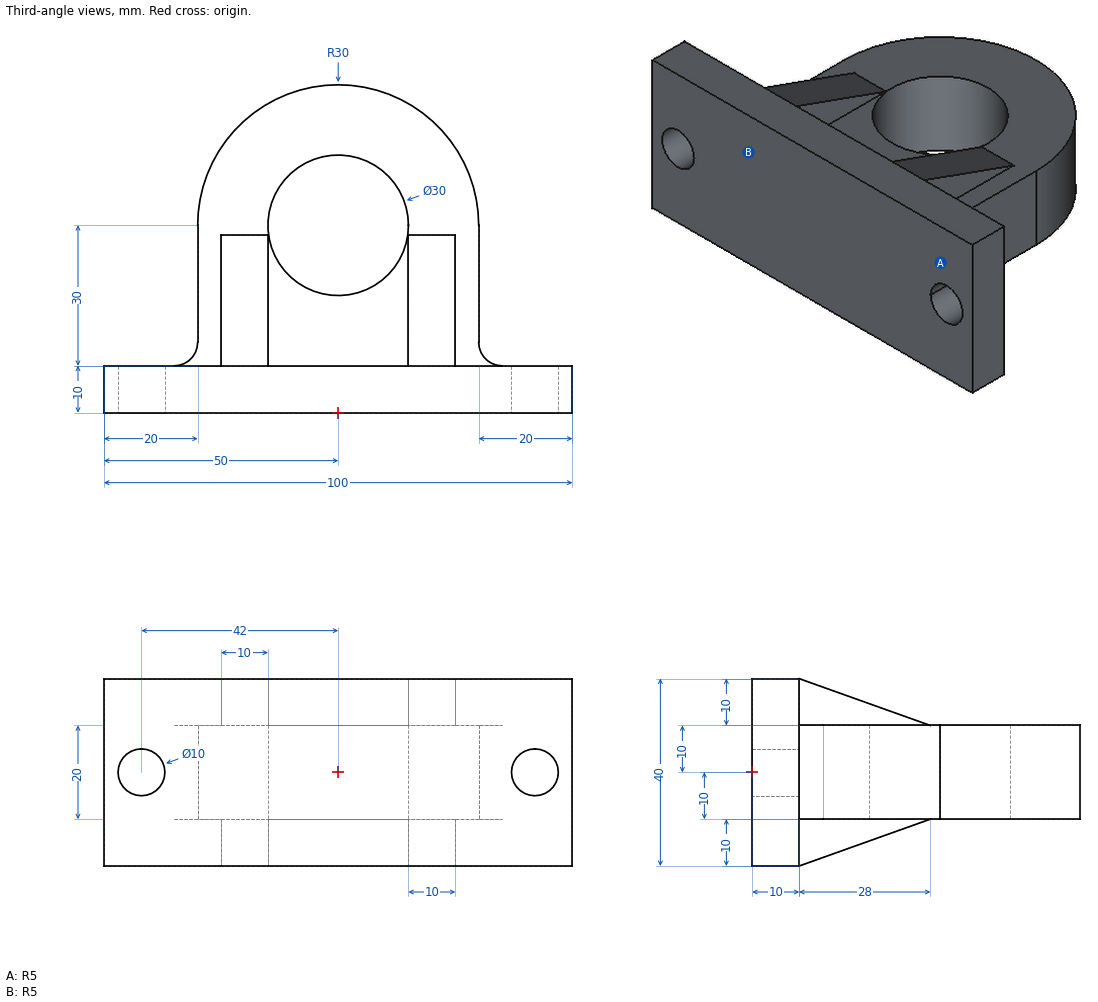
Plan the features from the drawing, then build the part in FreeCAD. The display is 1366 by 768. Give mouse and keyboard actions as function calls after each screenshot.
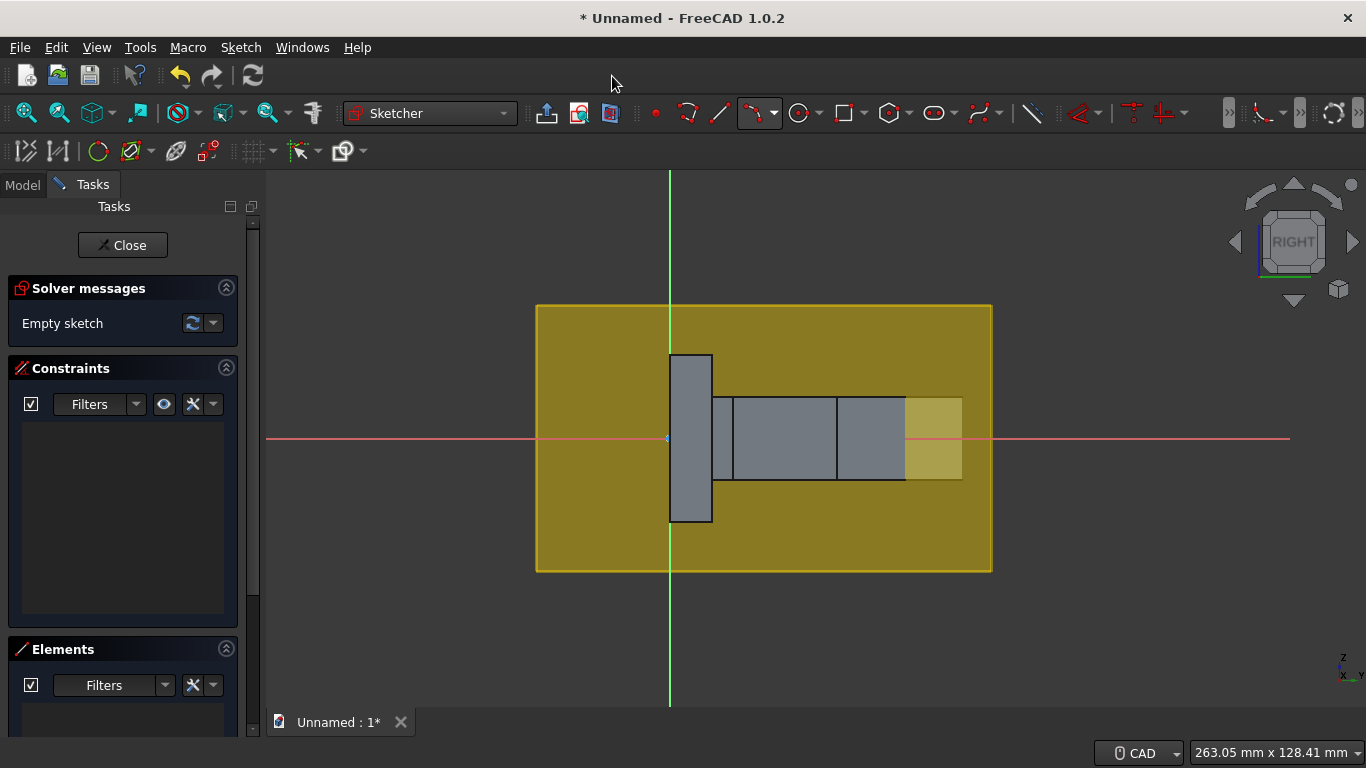
key(q)
key(s)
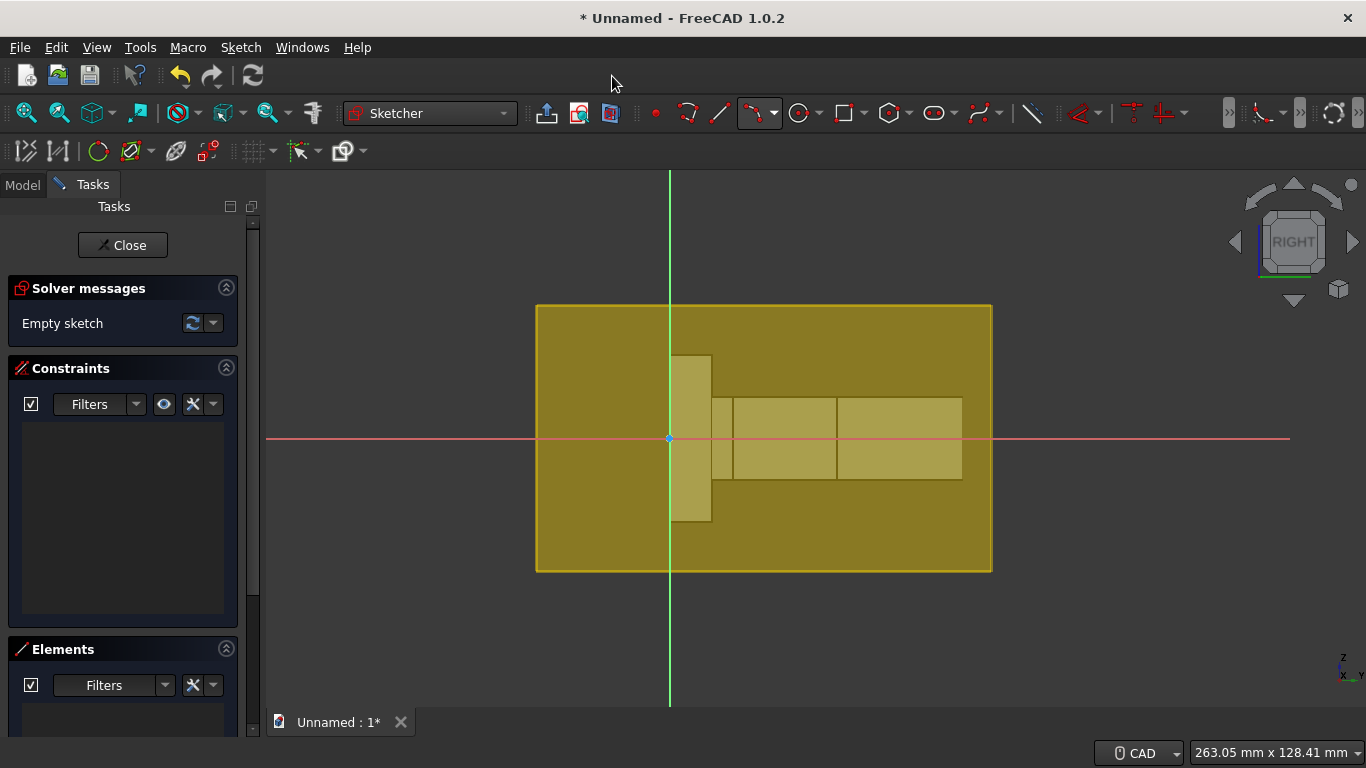
scroll(750, 494, up, 7)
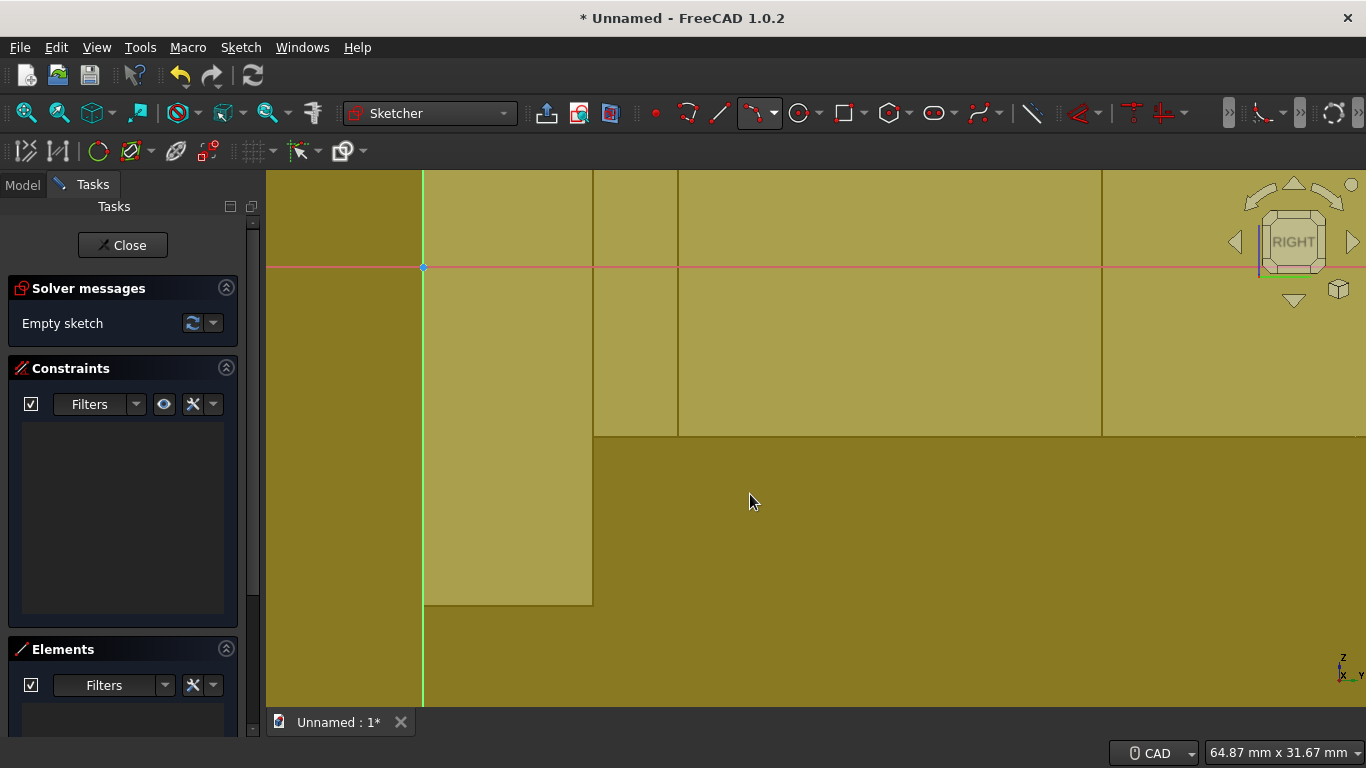
click(688, 114)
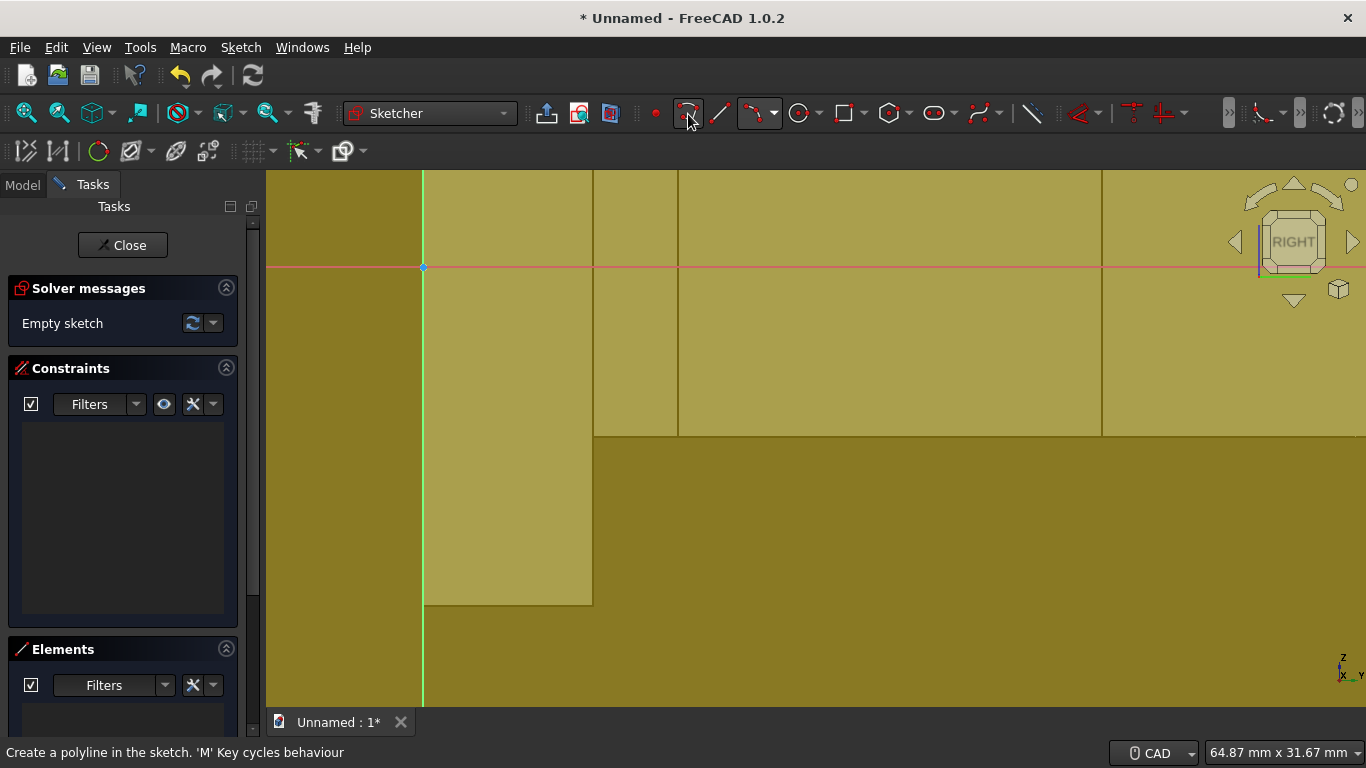
click(593, 437)
click(593, 606)
click(1068, 437)
click(593, 438)
key(Escape)
key(Escape)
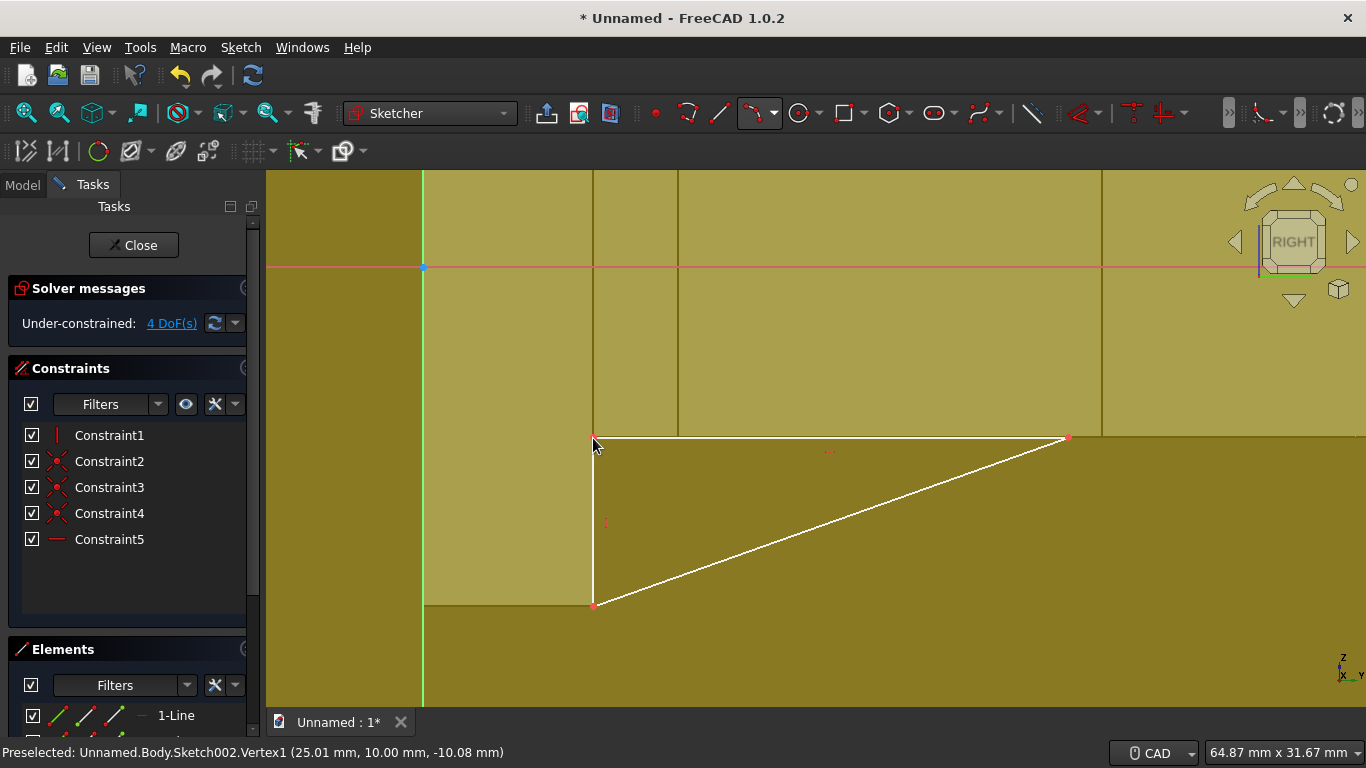
key(d)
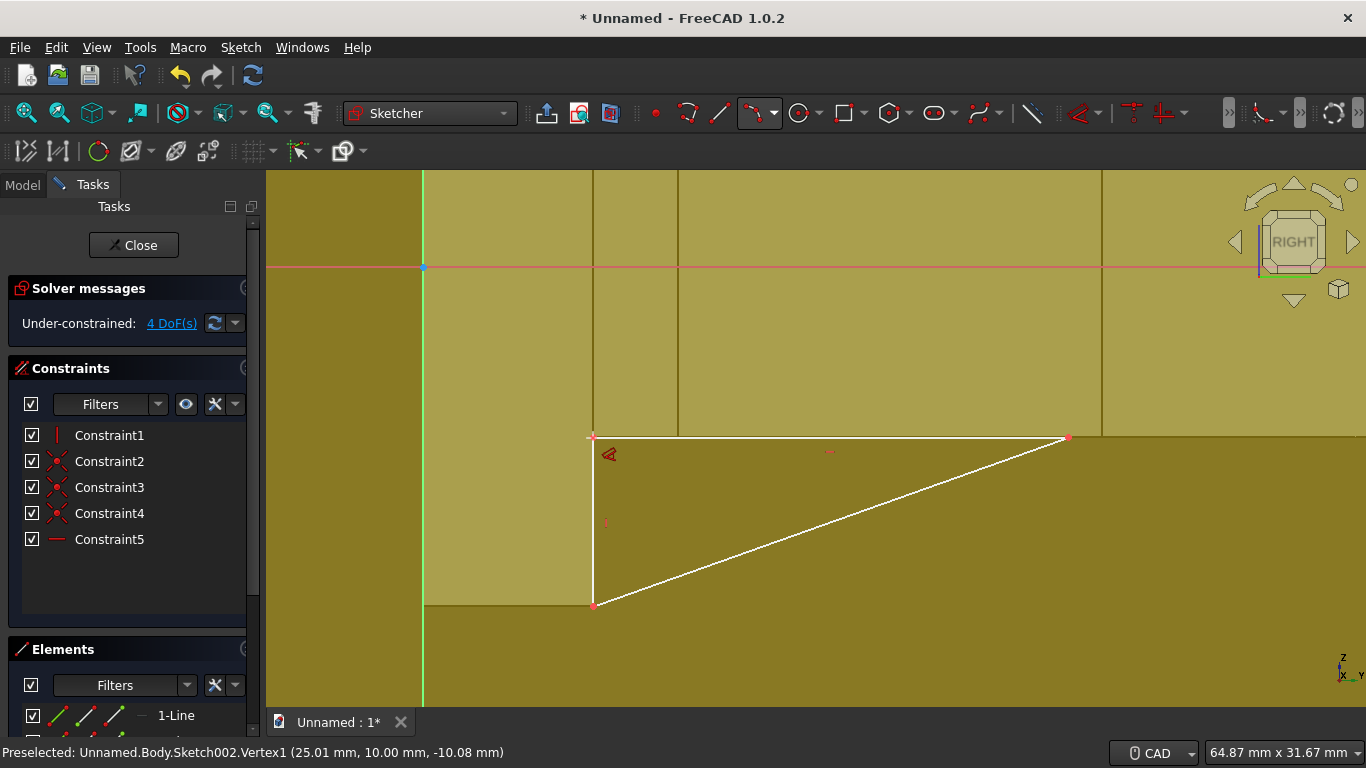
click(593, 489)
click(559, 523)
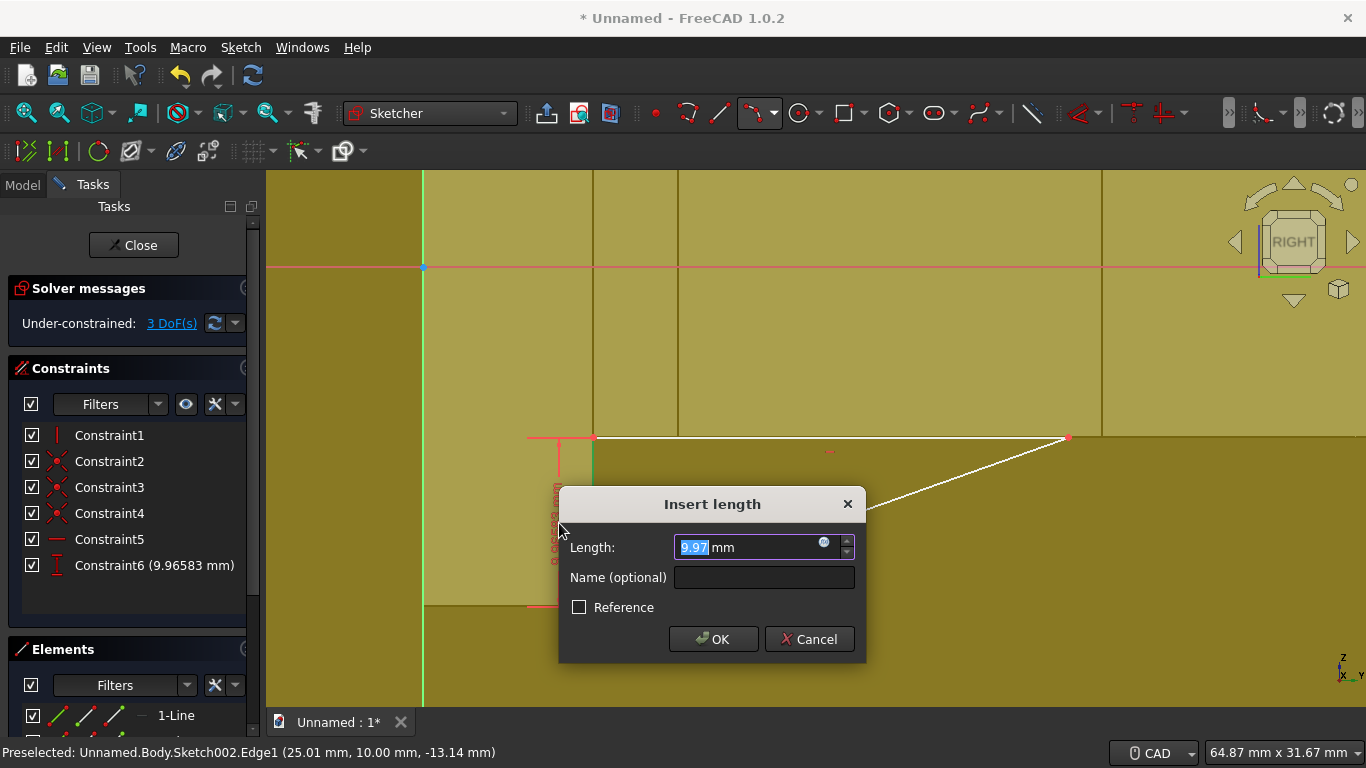
text(10)
key(Return)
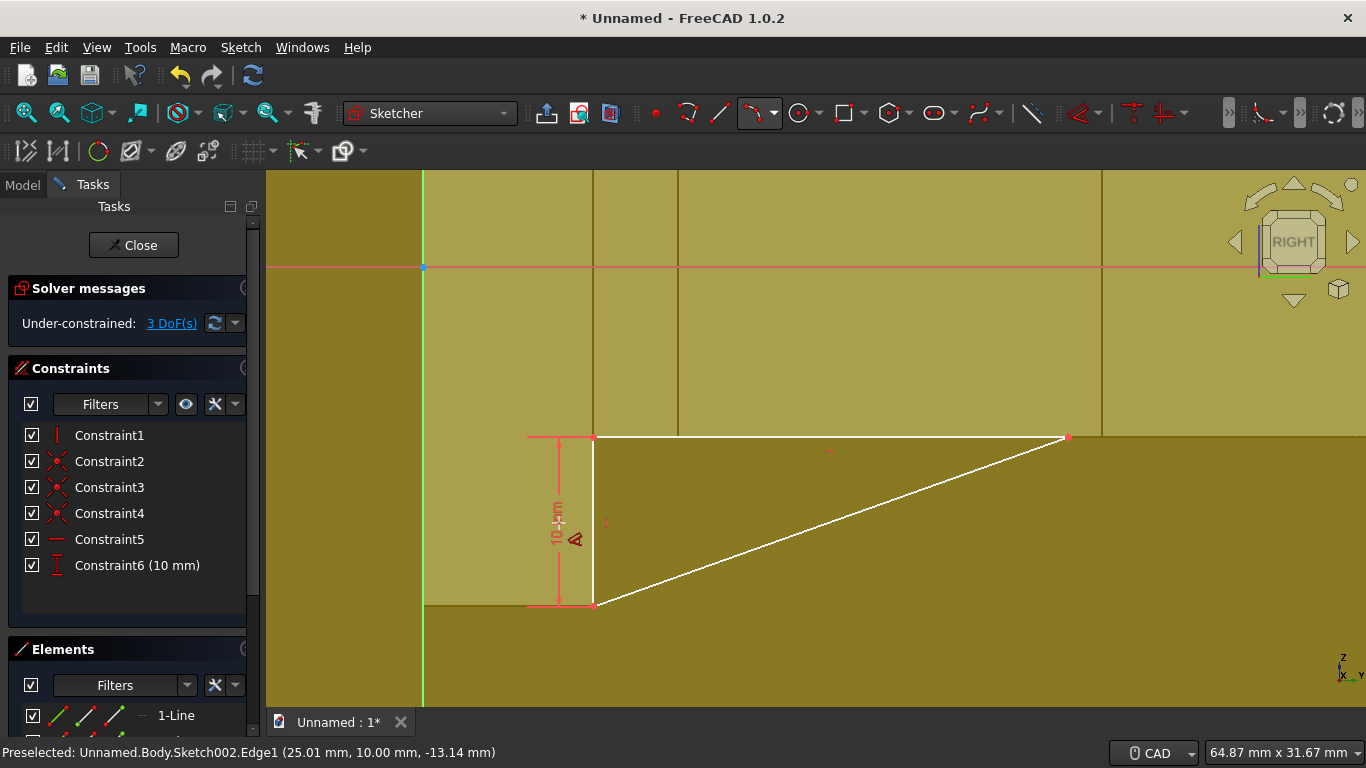
click(926, 437)
click(831, 471)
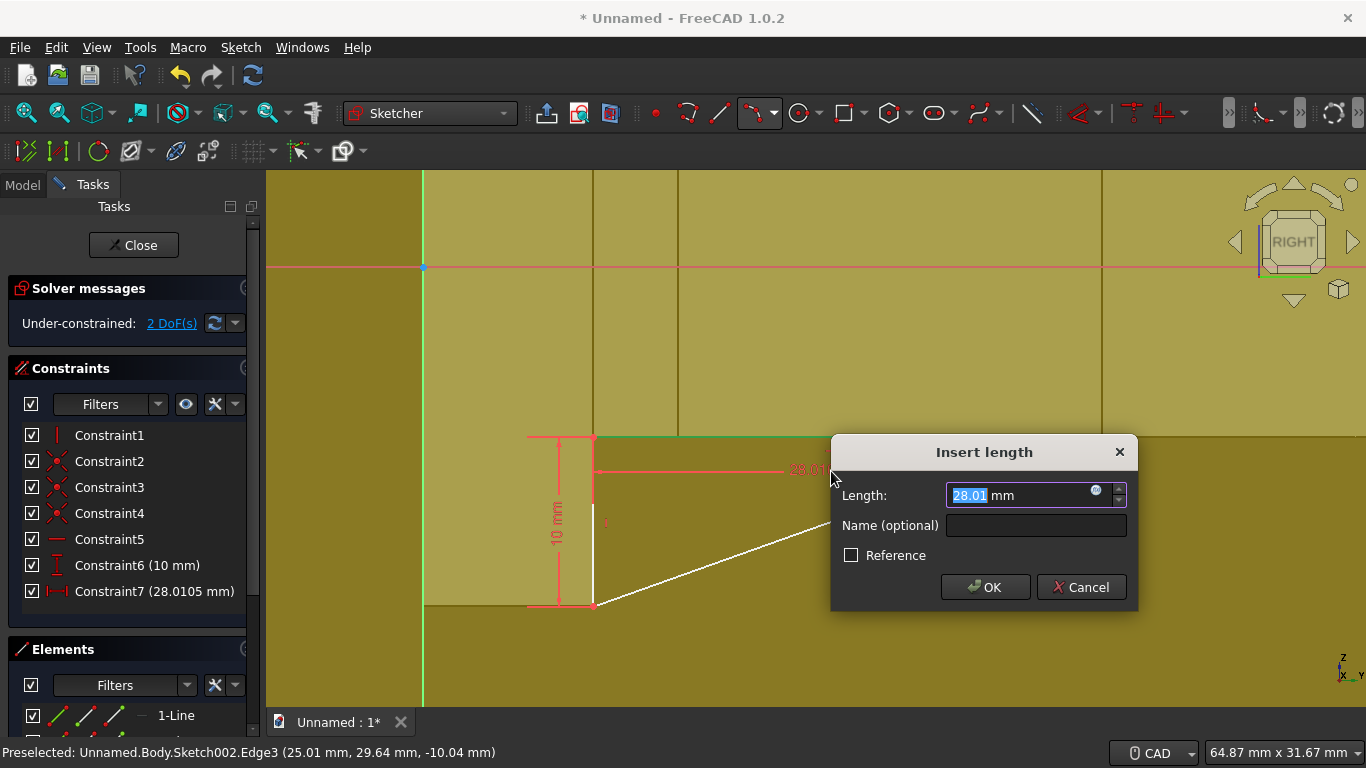
text(28)
key(Return)